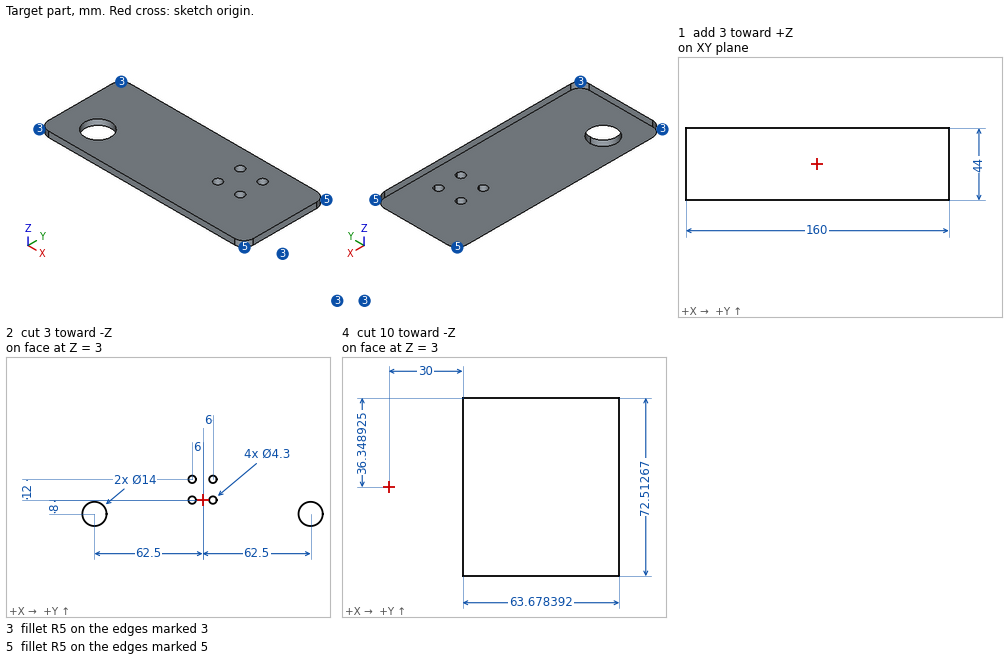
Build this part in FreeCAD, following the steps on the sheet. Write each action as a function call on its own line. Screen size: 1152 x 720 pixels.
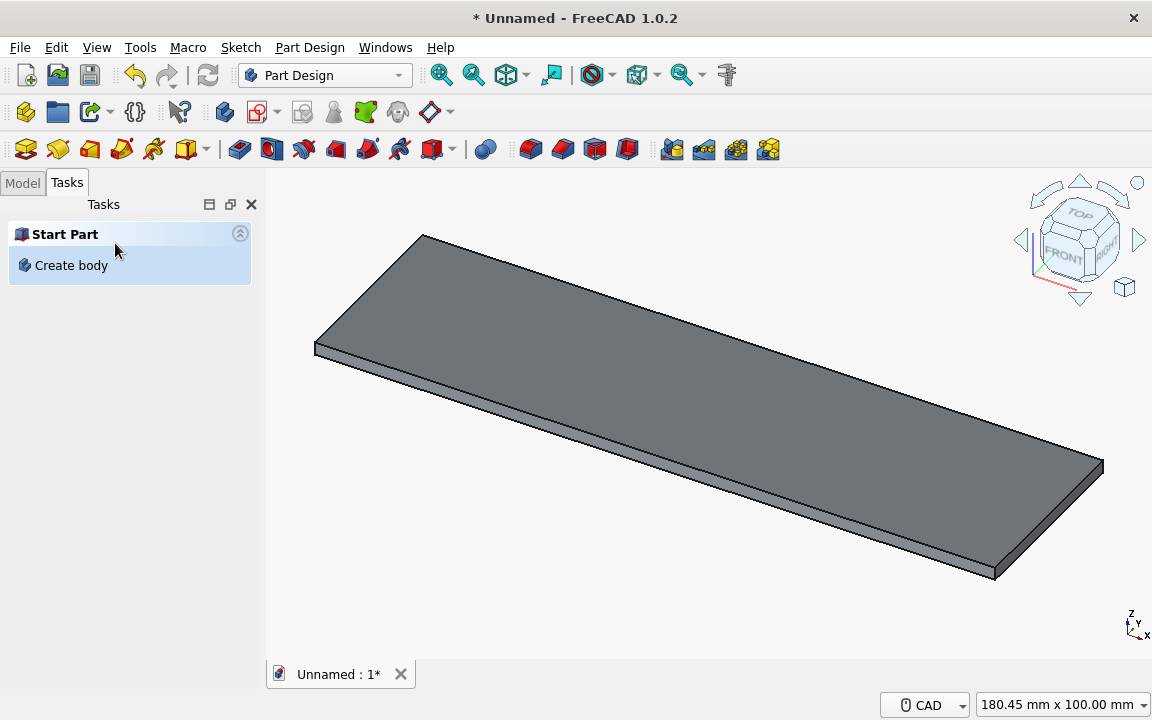
click(903, 465)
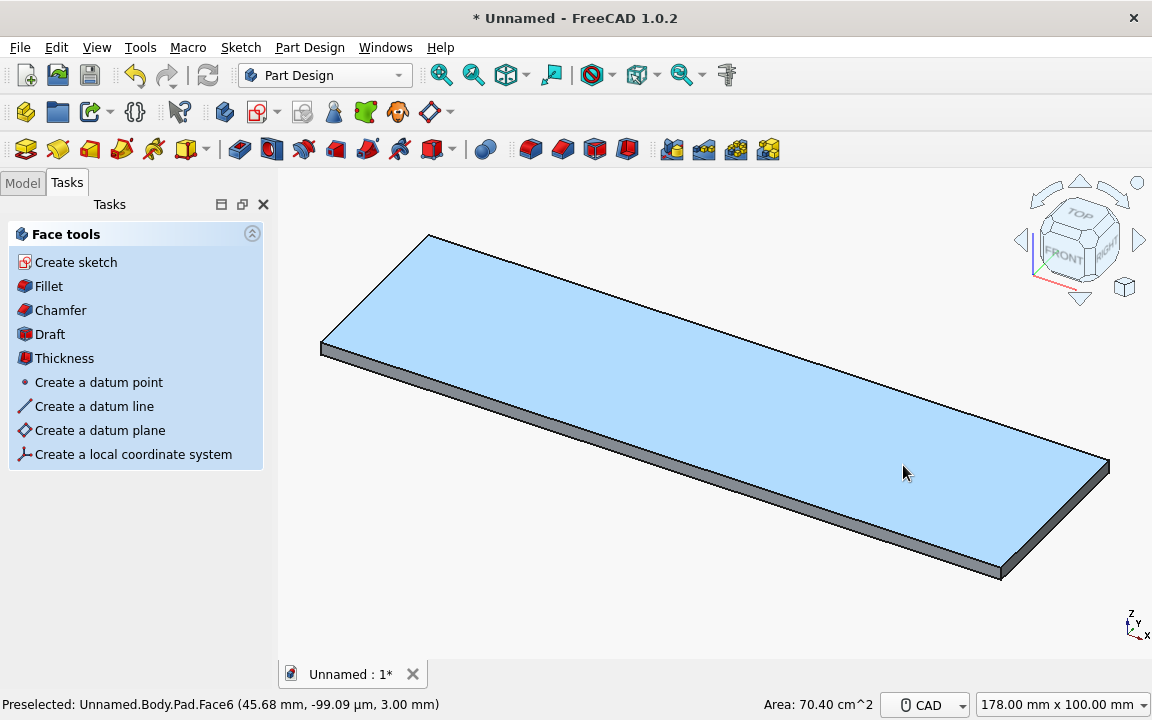
click(258, 112)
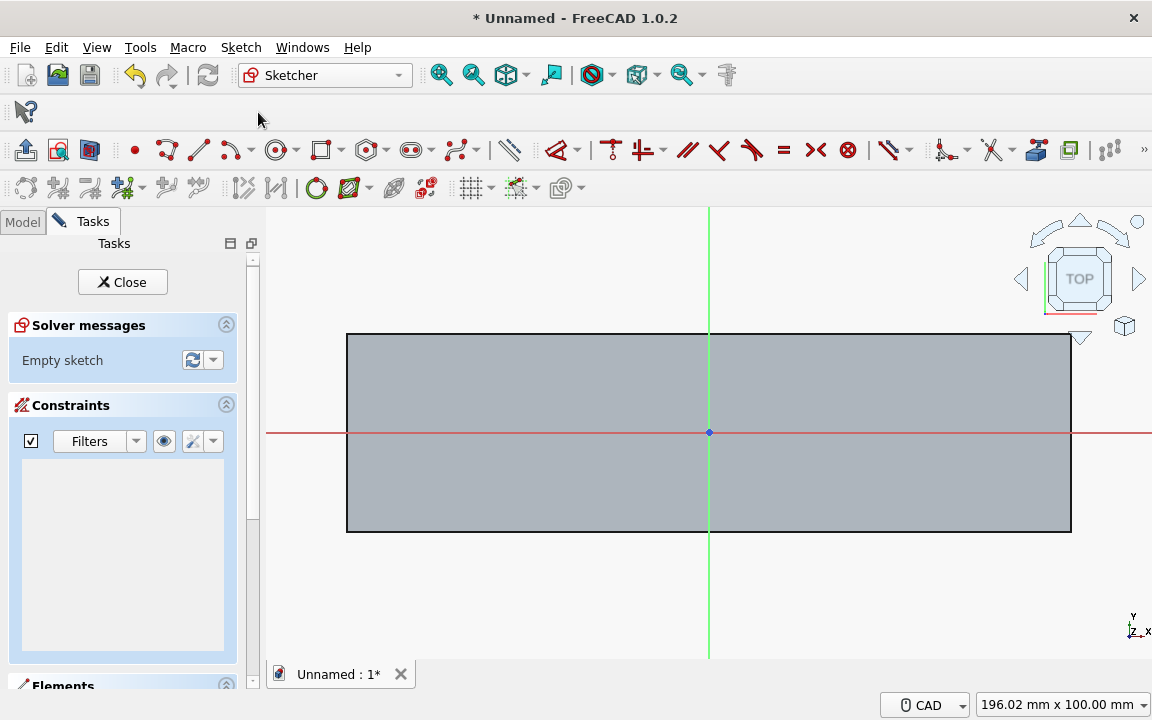
scroll(331, 424, down, 1)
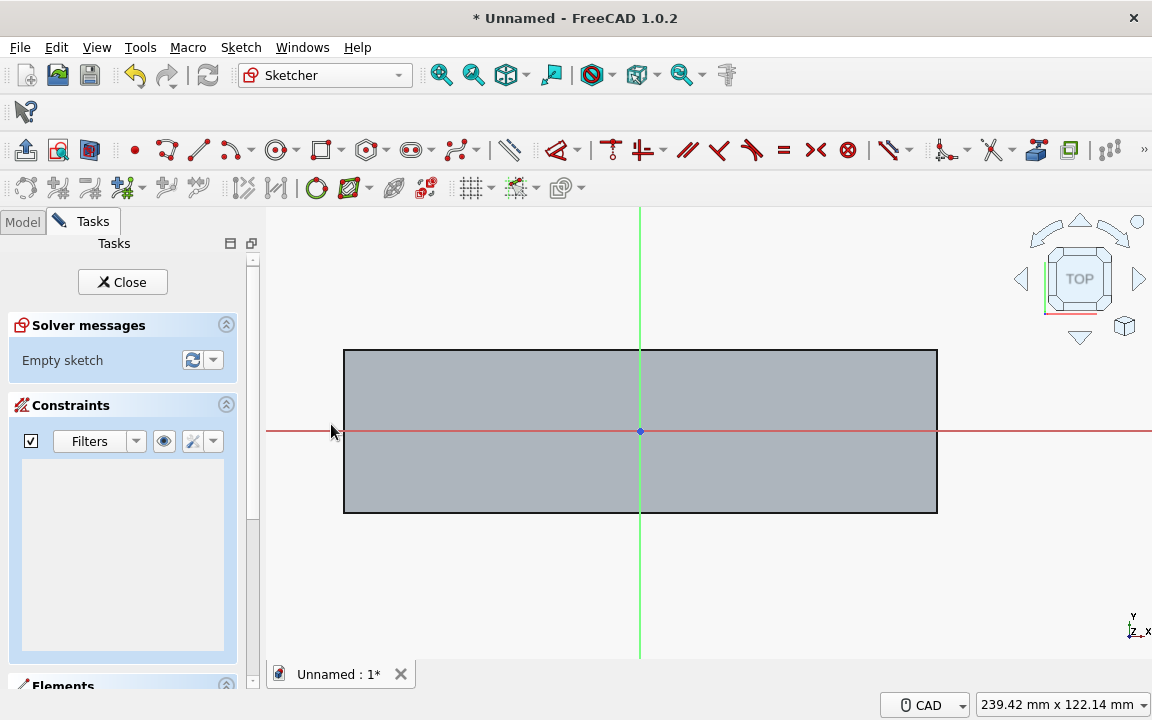
click(276, 150)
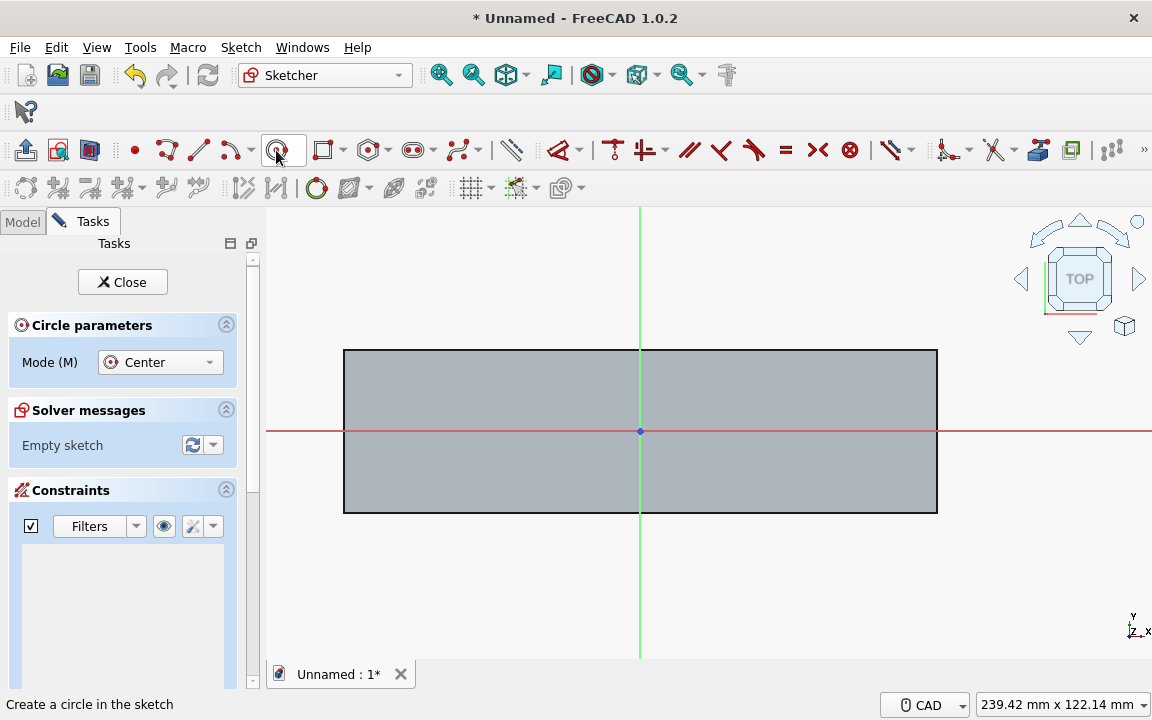
click(409, 461)
move(428, 479)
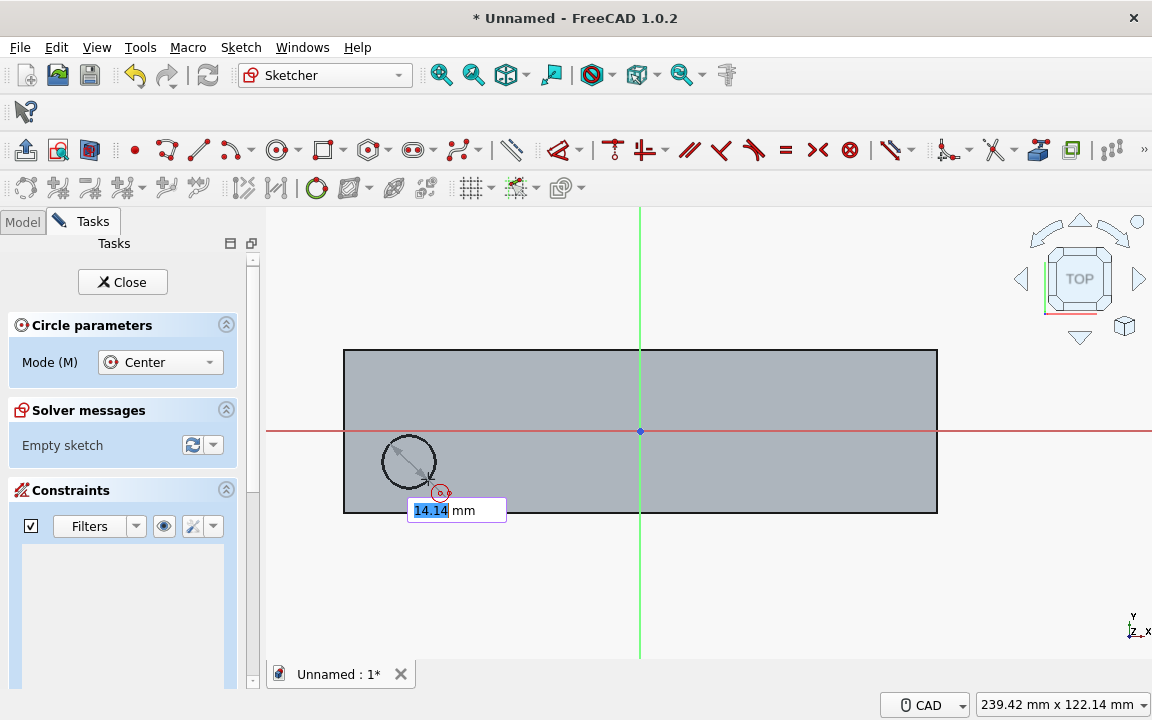
text(14)
key(Return)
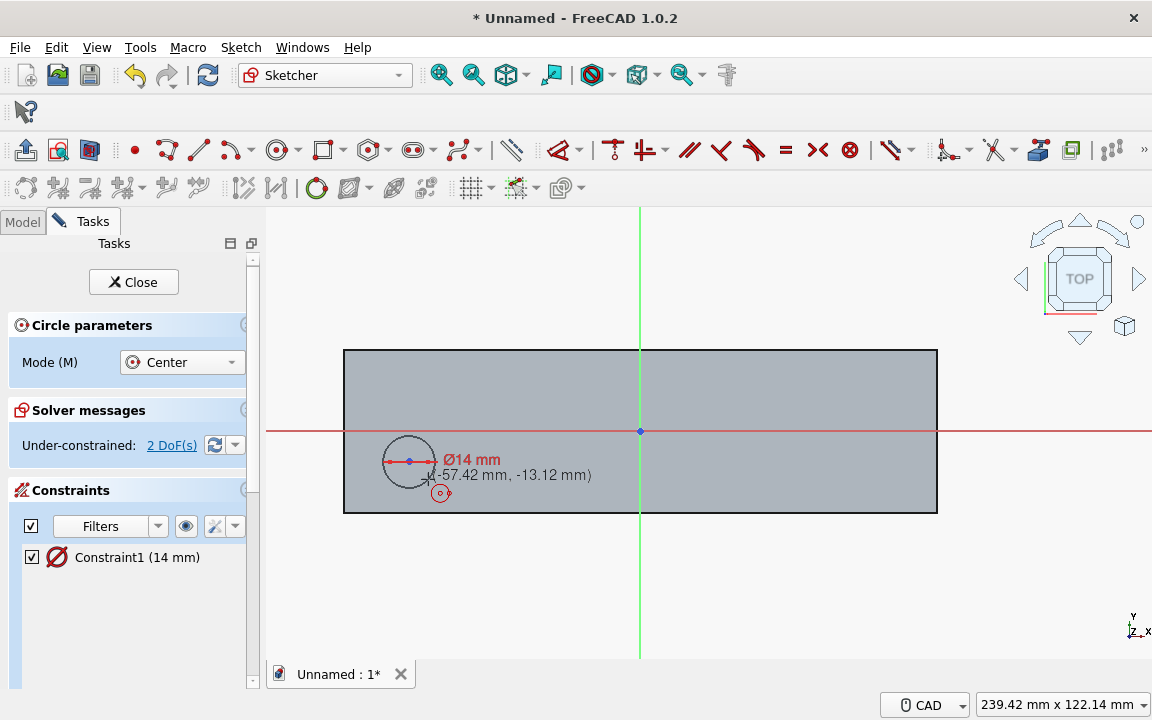
click(872, 461)
move(890, 479)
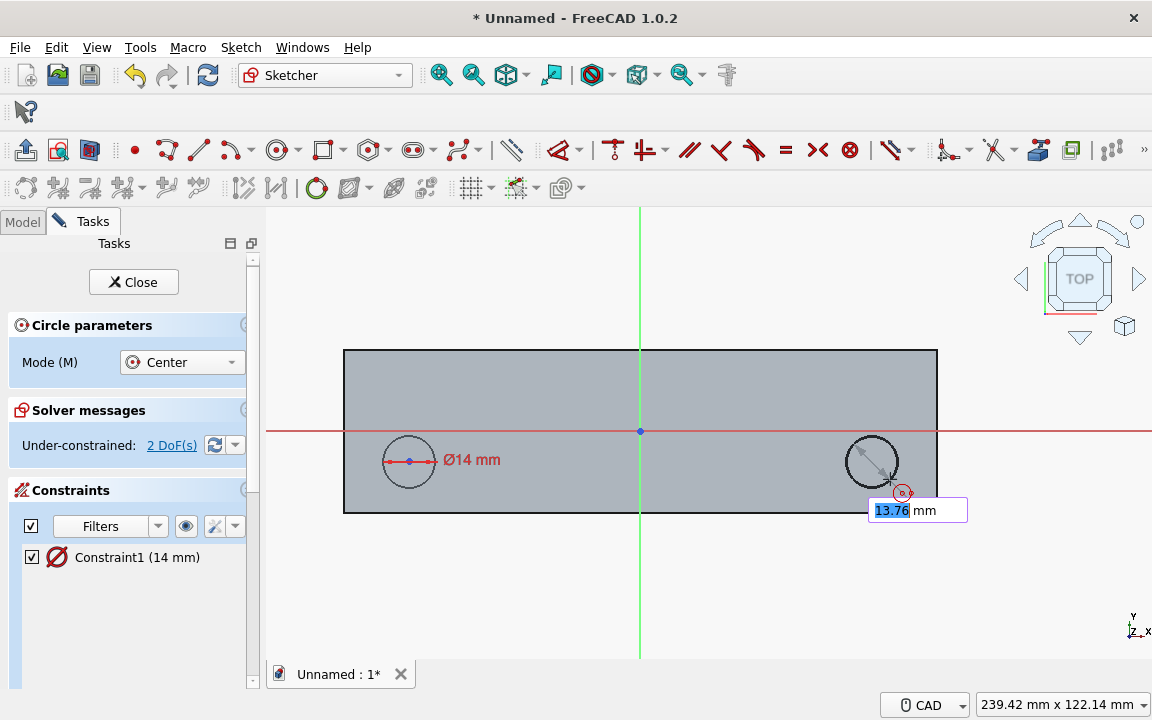
text(14)
key(Return)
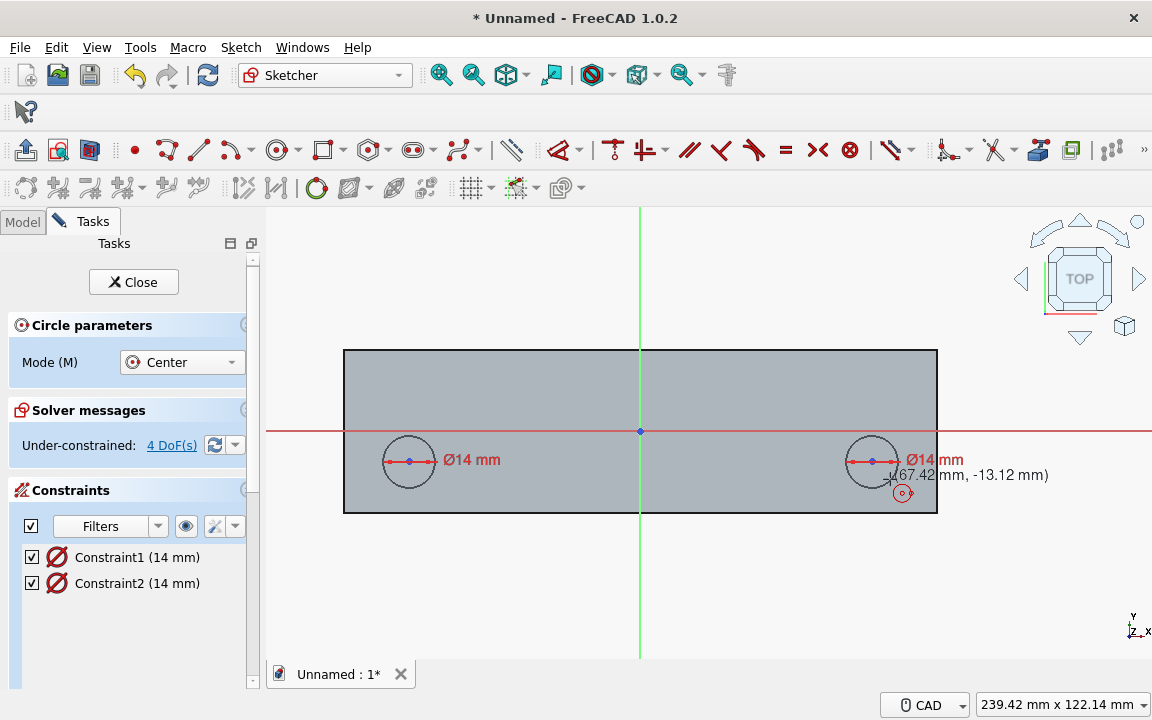
scroll(618, 387, up, 6)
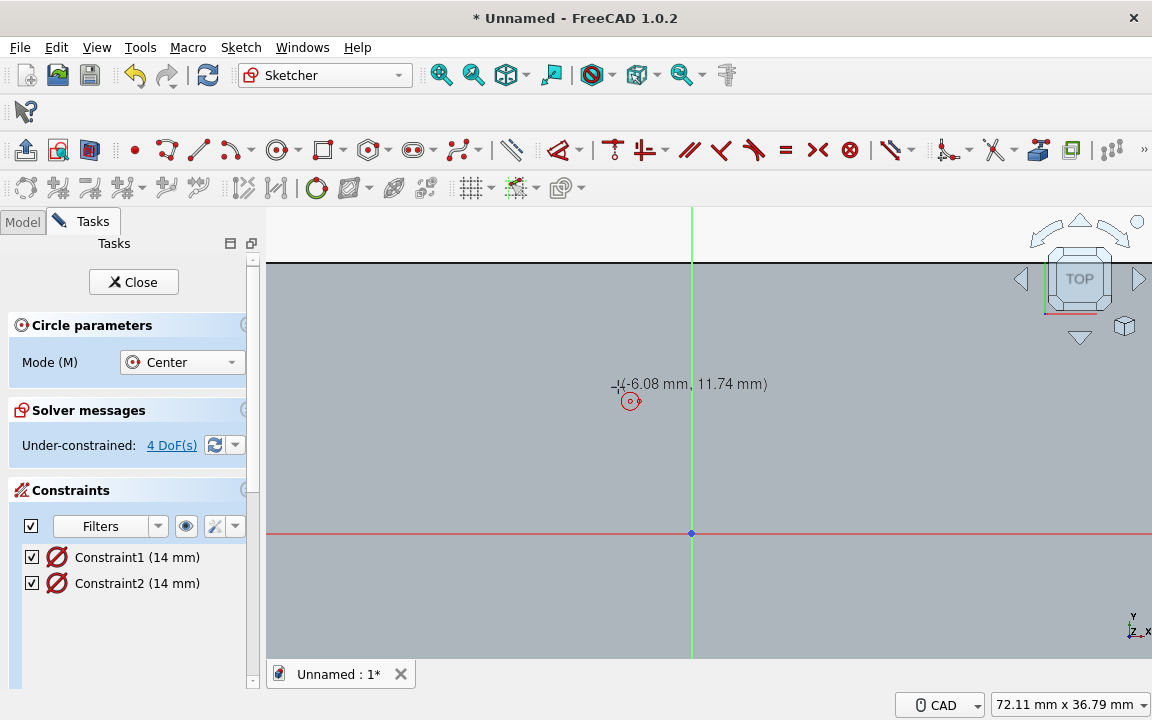
click(618, 386)
move(637, 368)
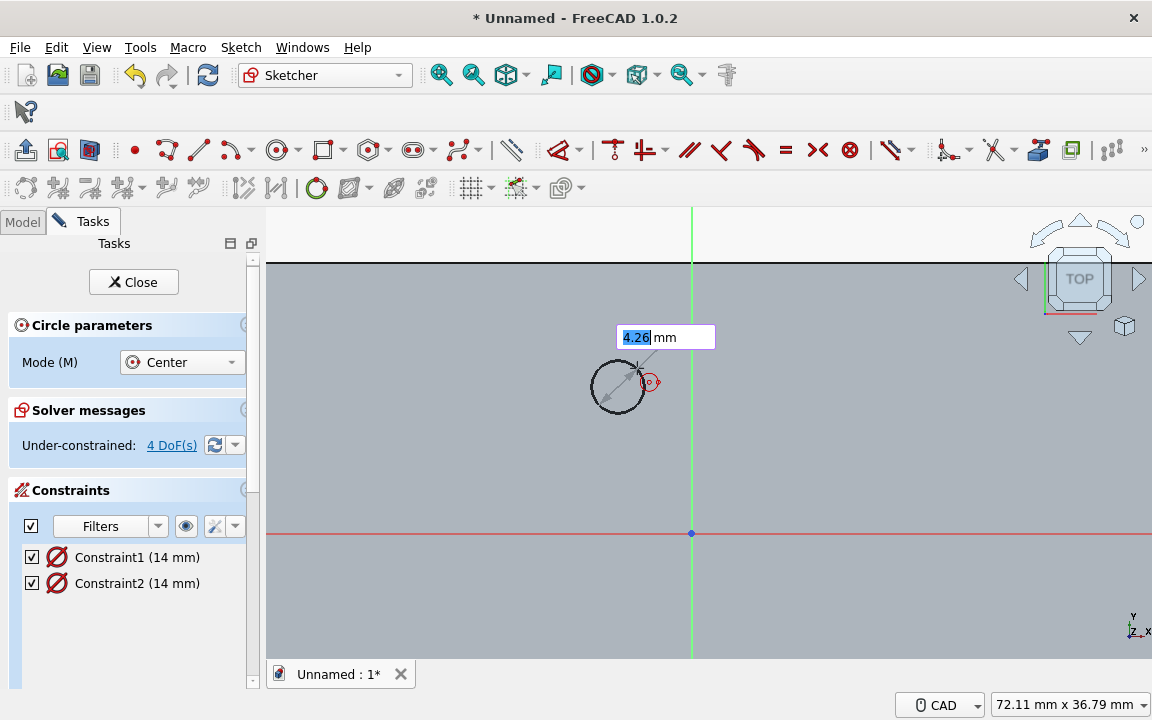
text(4.3)
key(Return)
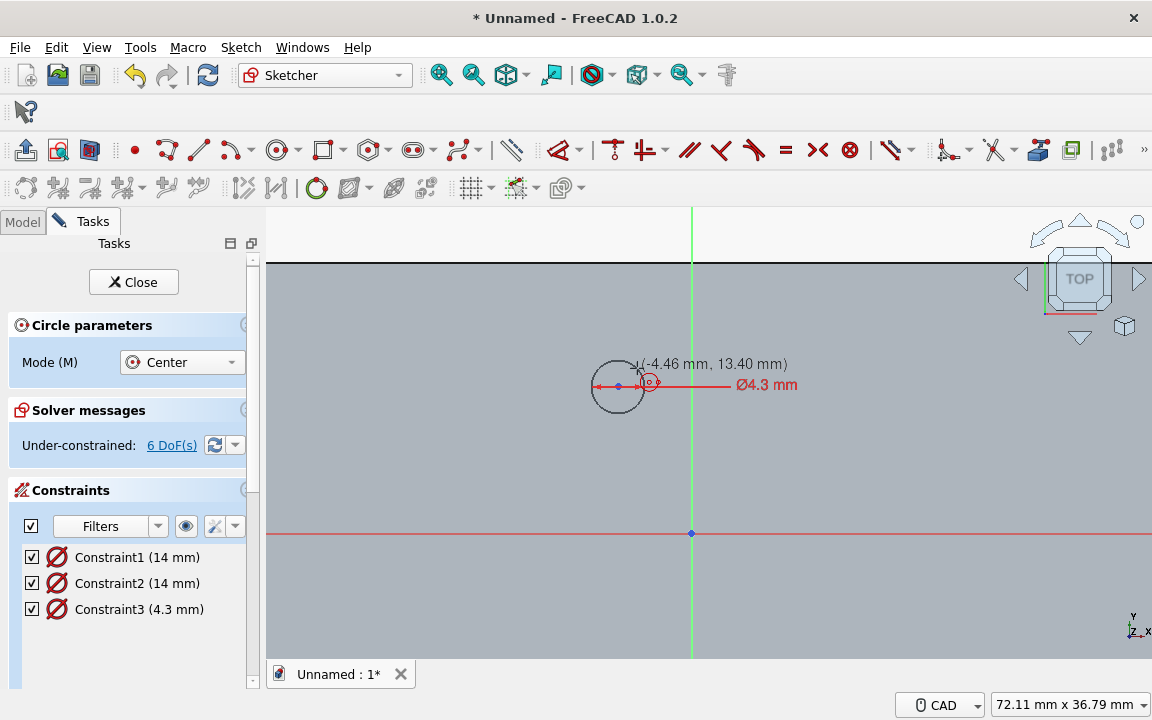
click(765, 386)
move(784, 368)